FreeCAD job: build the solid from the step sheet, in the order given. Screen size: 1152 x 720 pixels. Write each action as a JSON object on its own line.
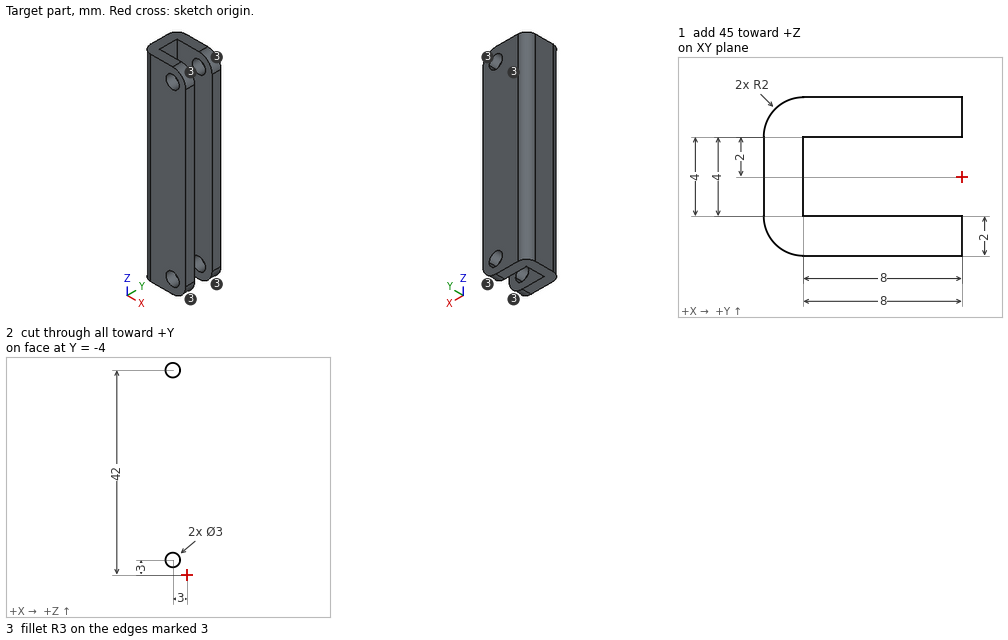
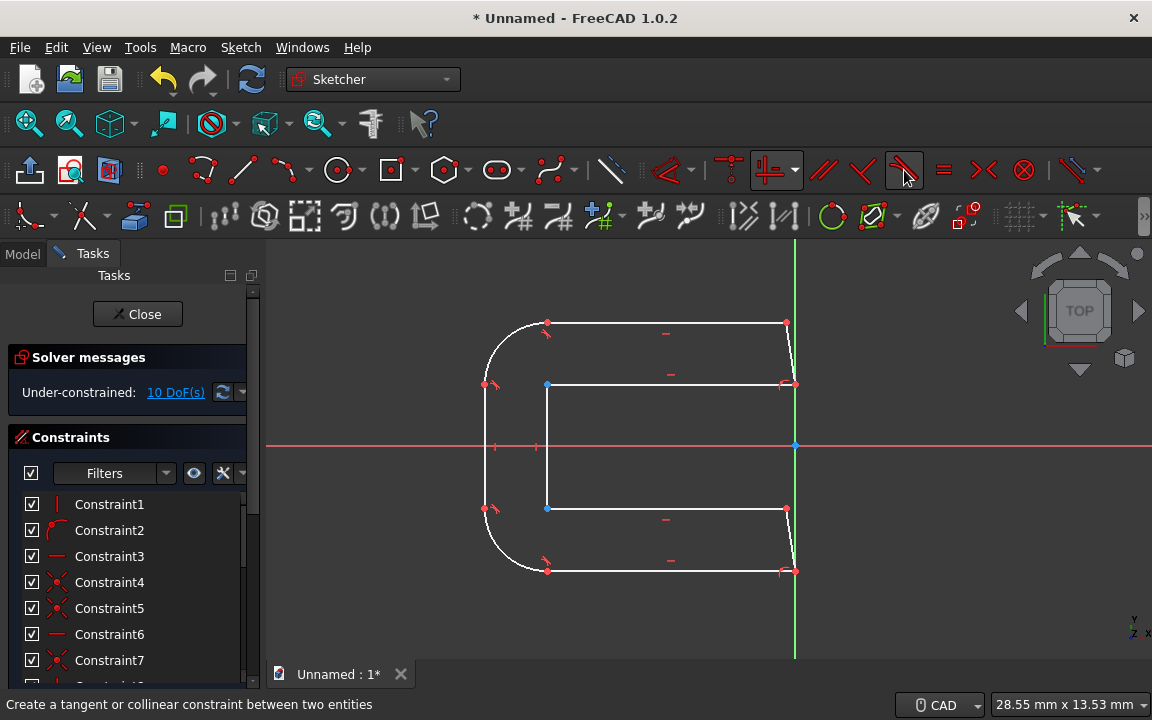
{"action": "left_click", "coordinate": [793, 552]}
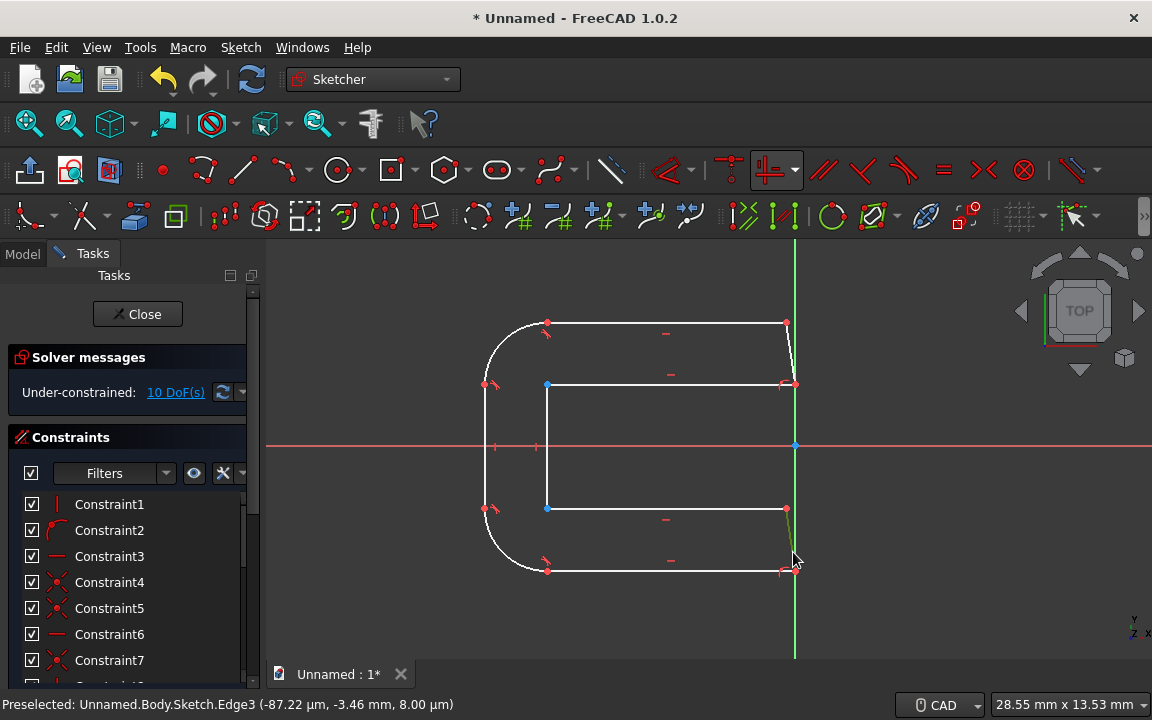
{"action": "key", "text": "v"}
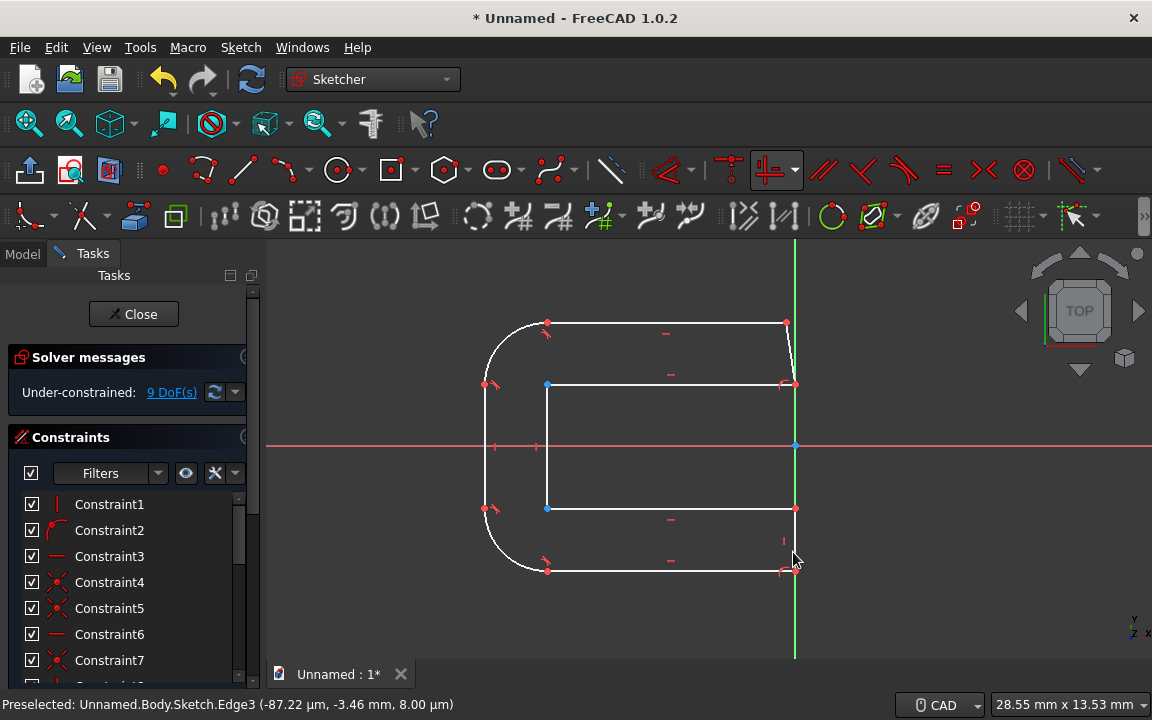
{"action": "left_click", "coordinate": [793, 366]}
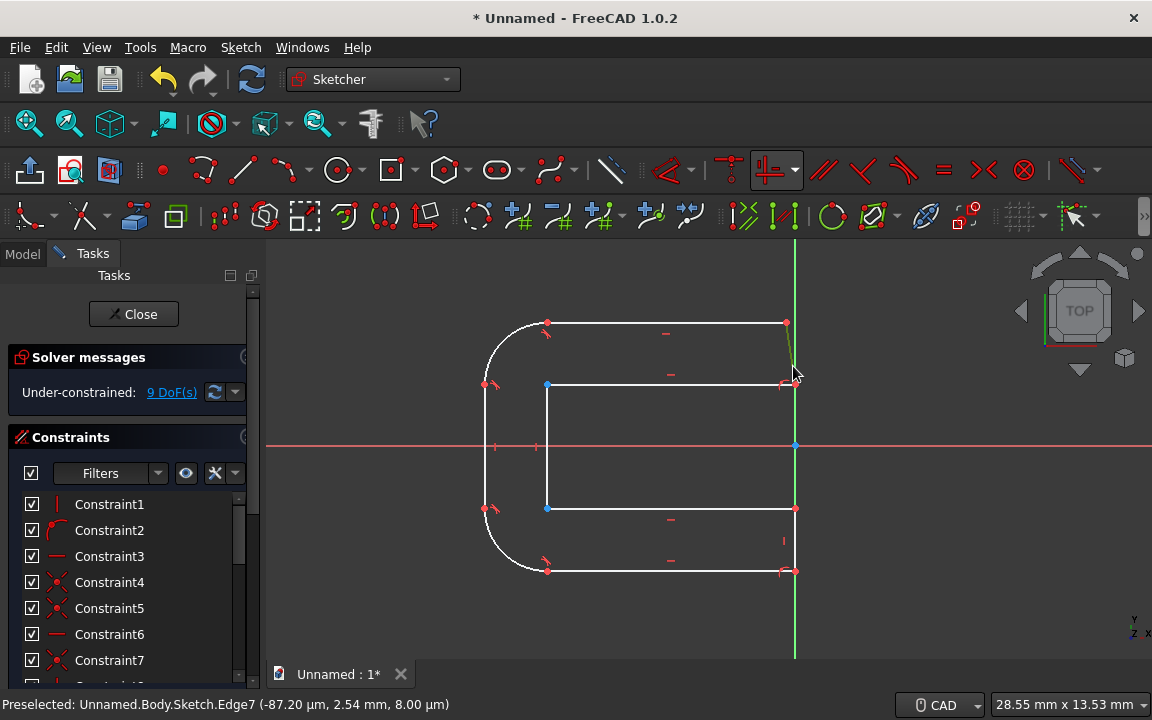
{"action": "left_click", "coordinate": [798, 170]}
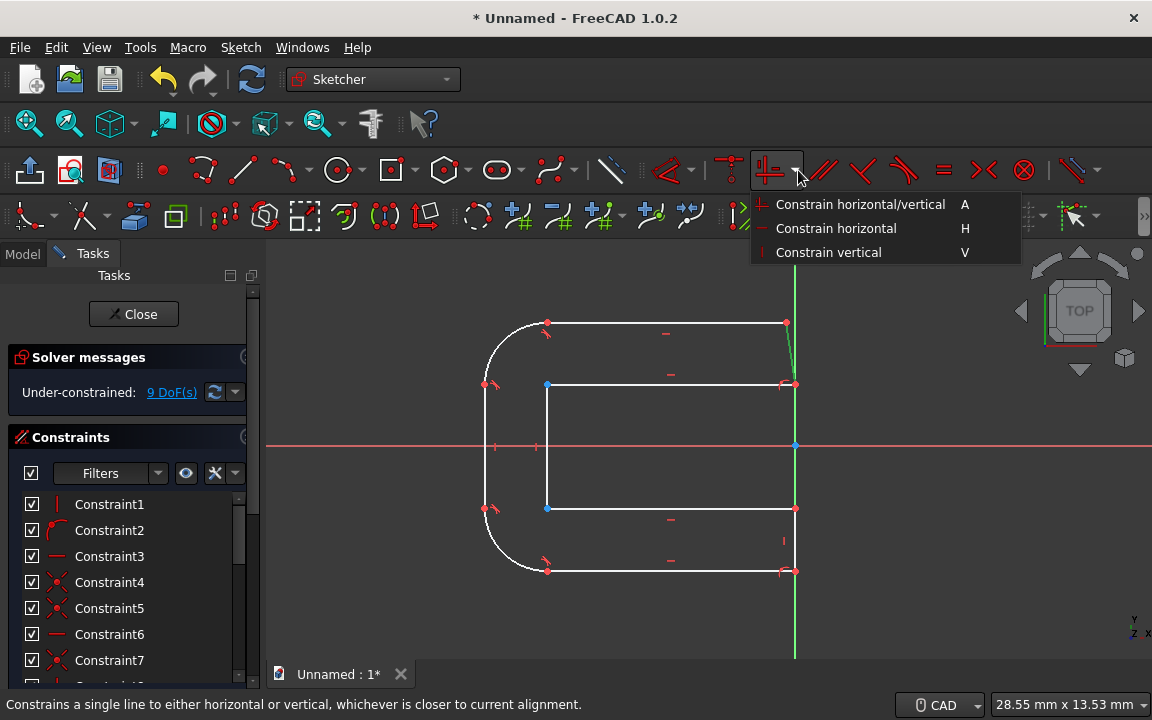
{"action": "left_click", "coordinate": [886, 252]}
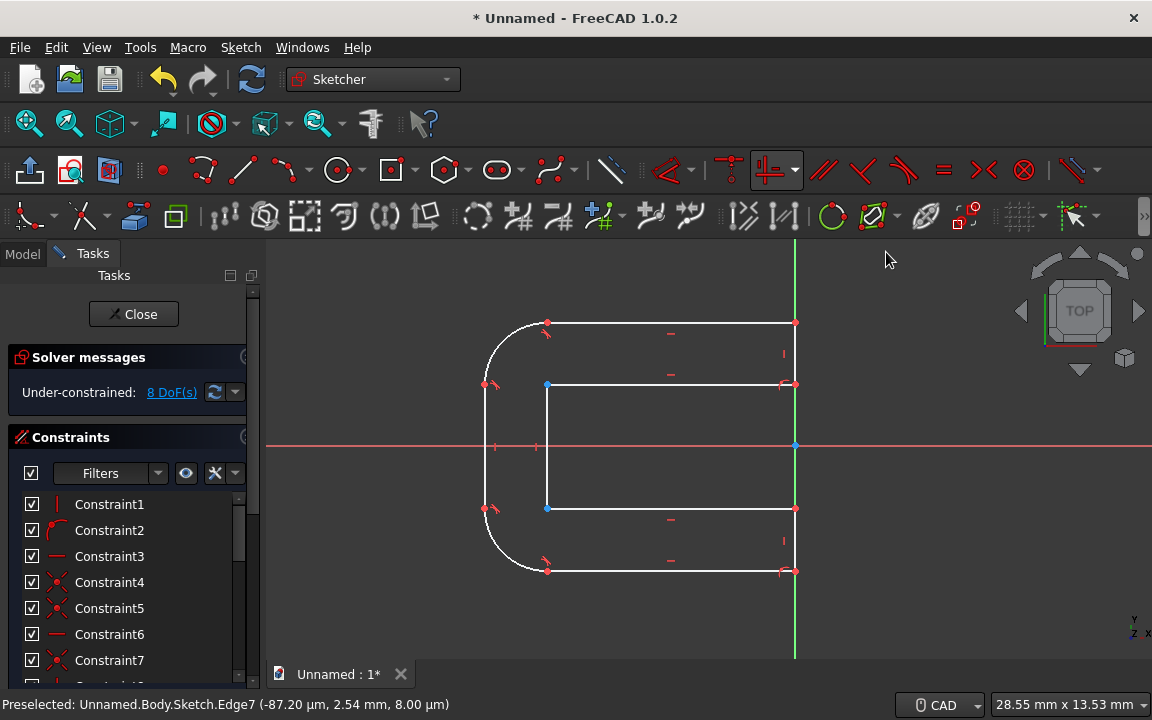
{"action": "left_click", "coordinate": [492, 537]}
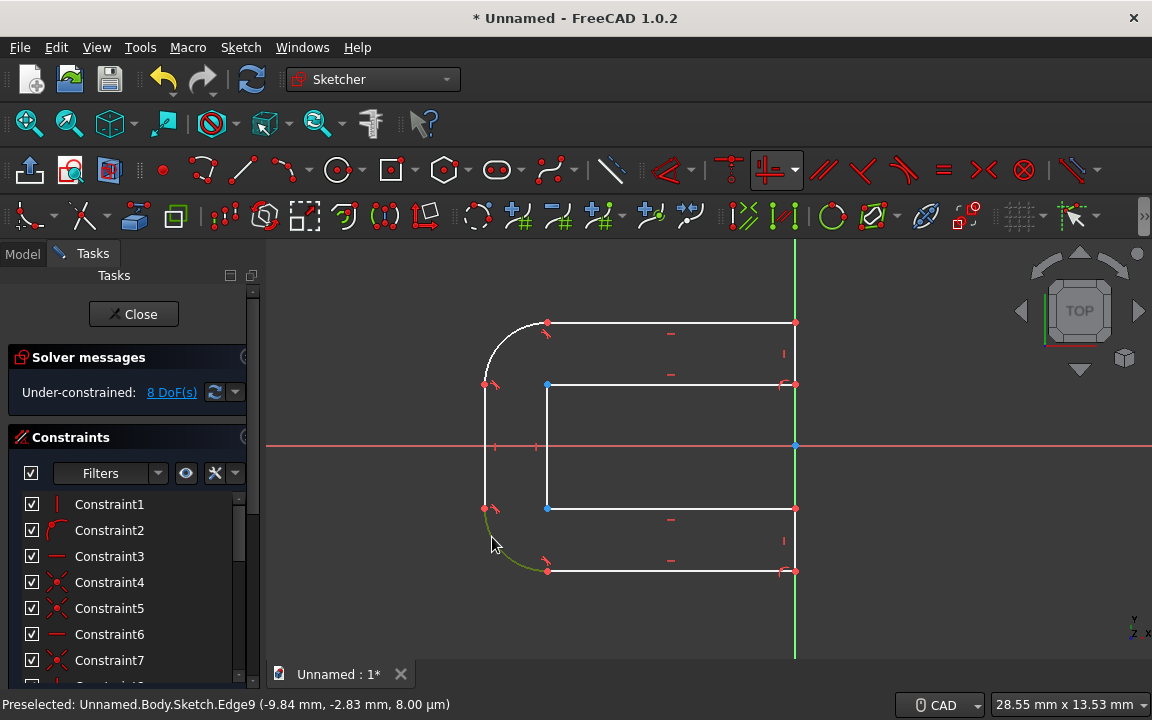
{"action": "left_click", "coordinate": [519, 330]}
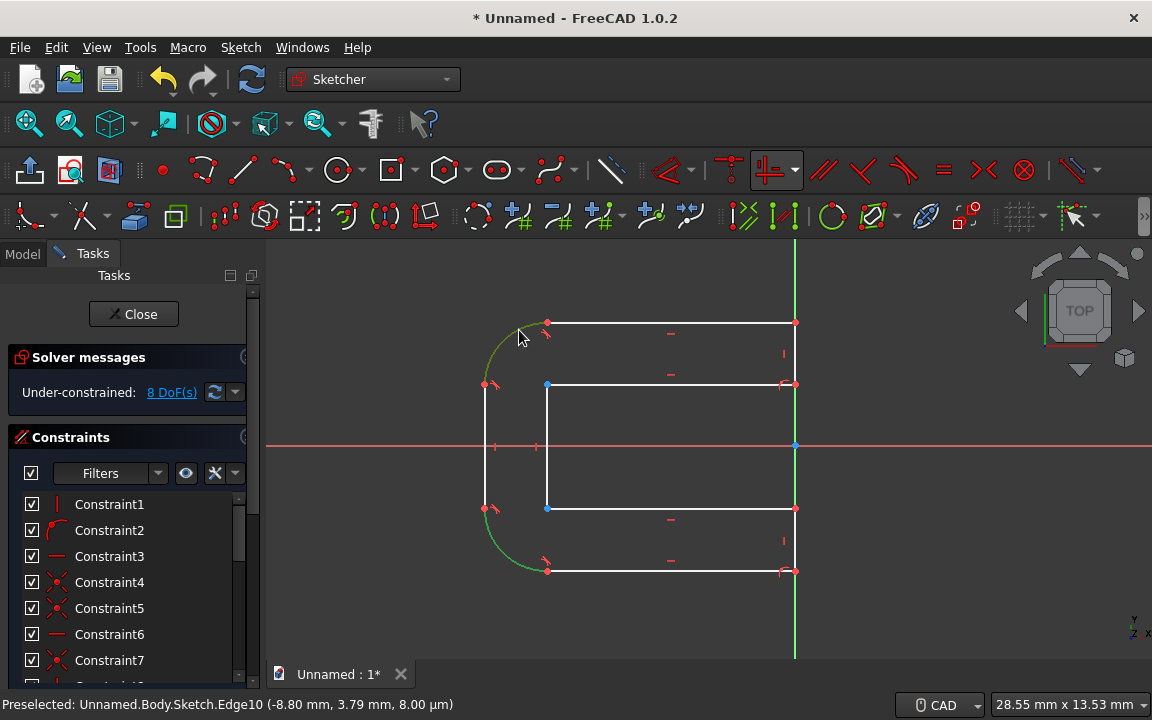
{"action": "left_click", "coordinate": [944, 170]}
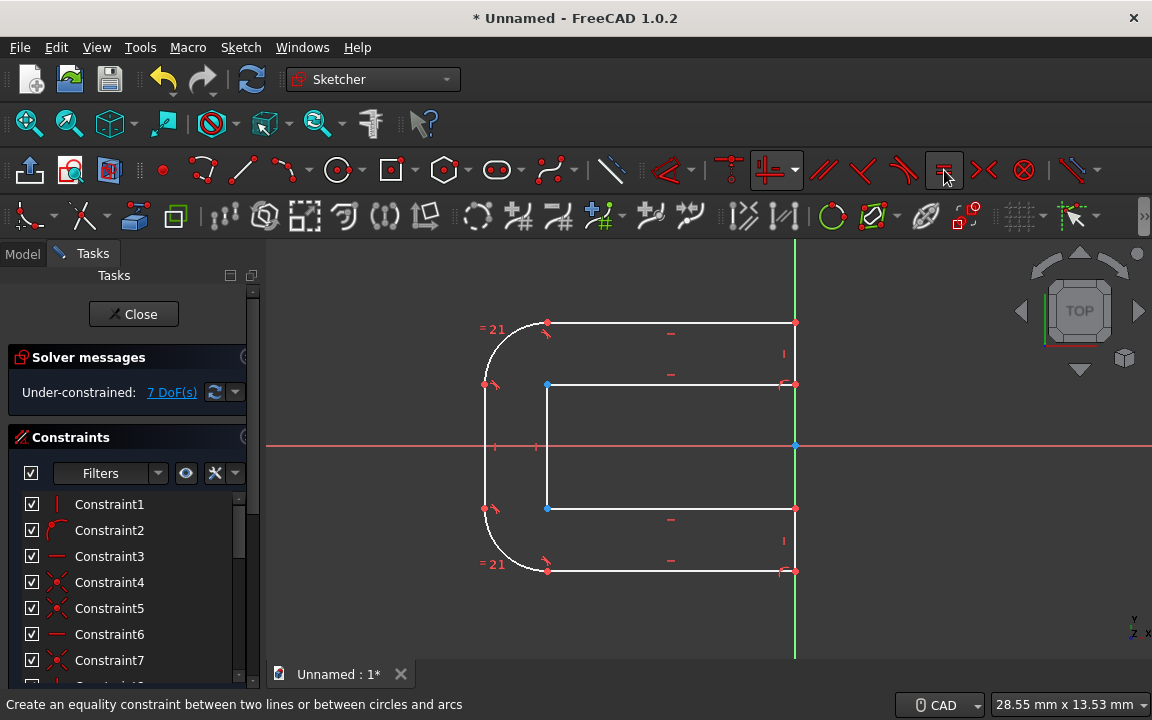
{"action": "left_click", "coordinate": [666, 170]}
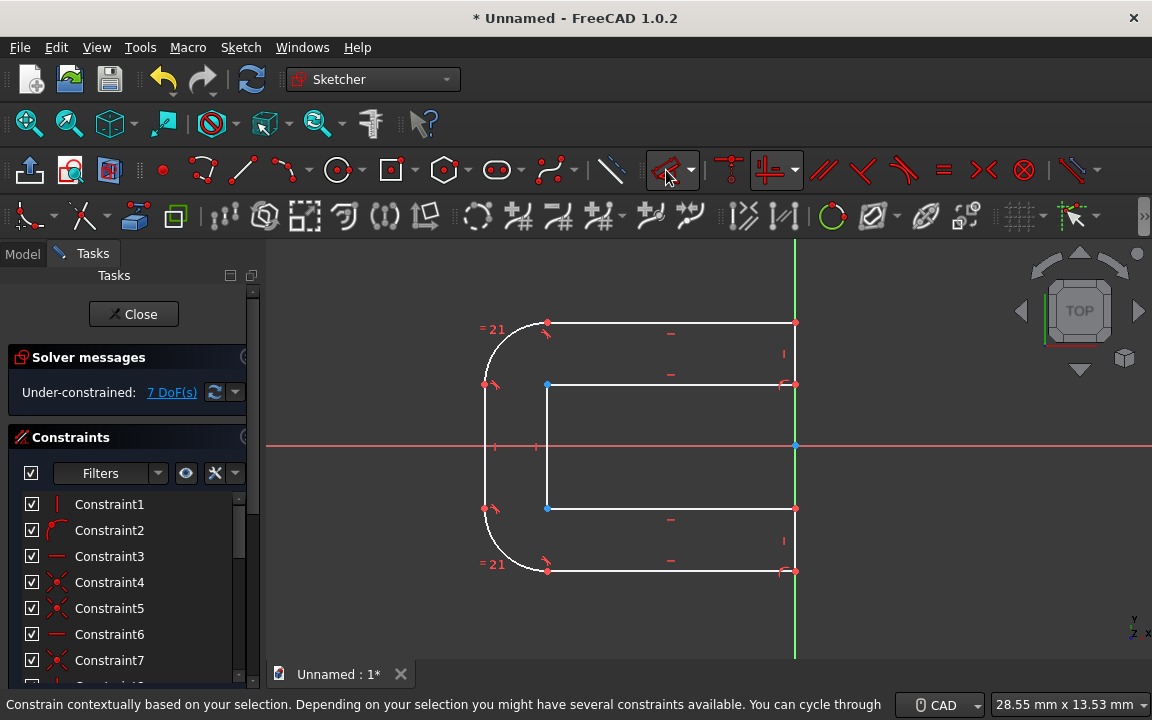
{"action": "left_click", "coordinate": [492, 537]}
{"action": "left_click", "coordinate": [463, 552]}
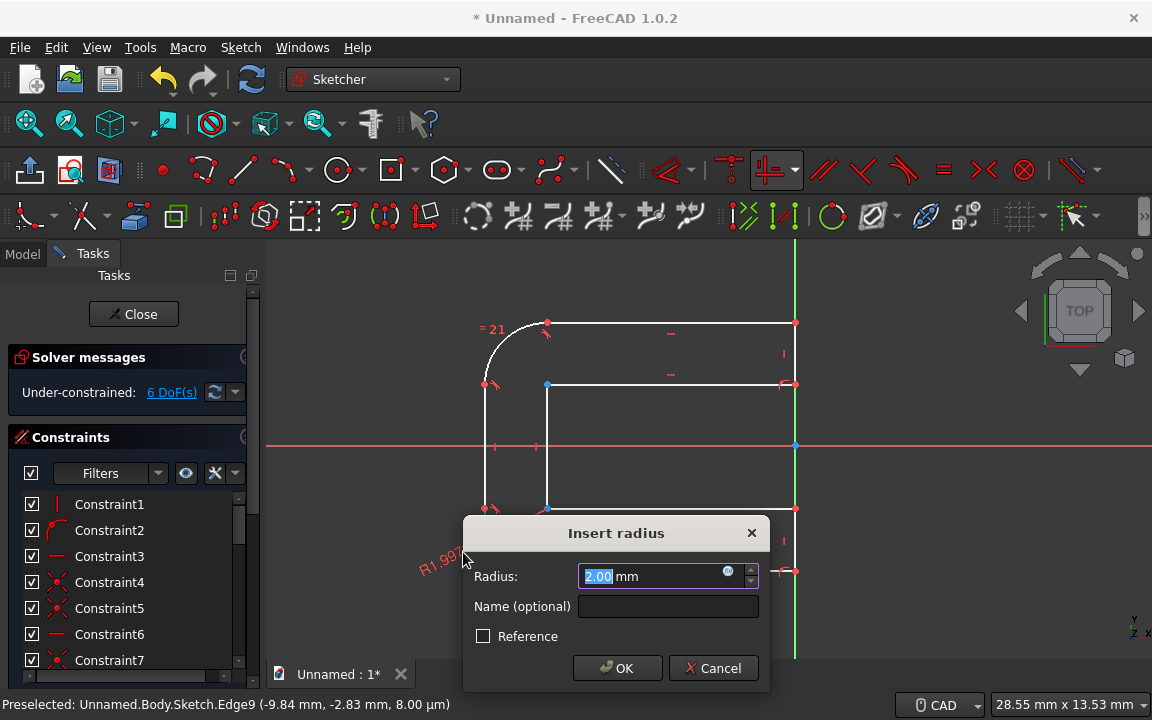
{"action": "type", "text": "2"}
{"action": "key", "text": "Return"}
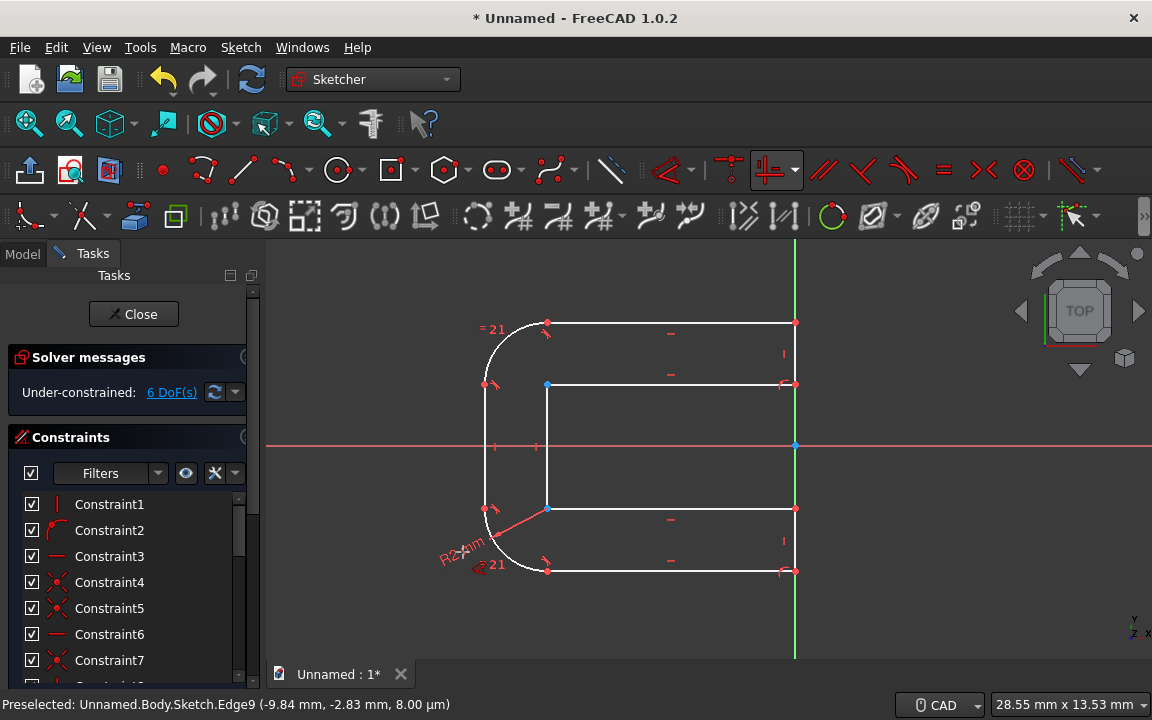
{"action": "left_click", "coordinate": [485, 422]}
{"action": "left_click", "coordinate": [451, 418]}